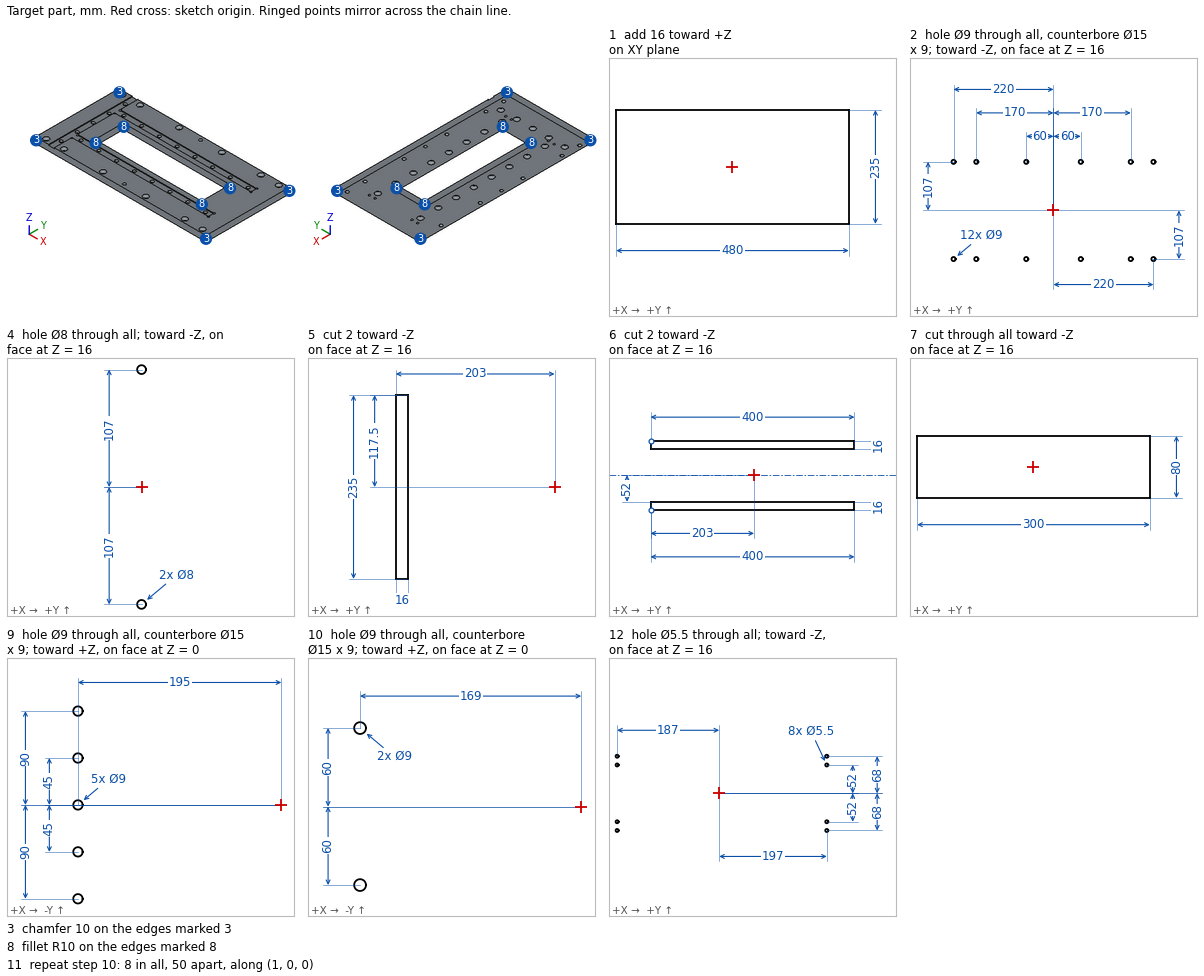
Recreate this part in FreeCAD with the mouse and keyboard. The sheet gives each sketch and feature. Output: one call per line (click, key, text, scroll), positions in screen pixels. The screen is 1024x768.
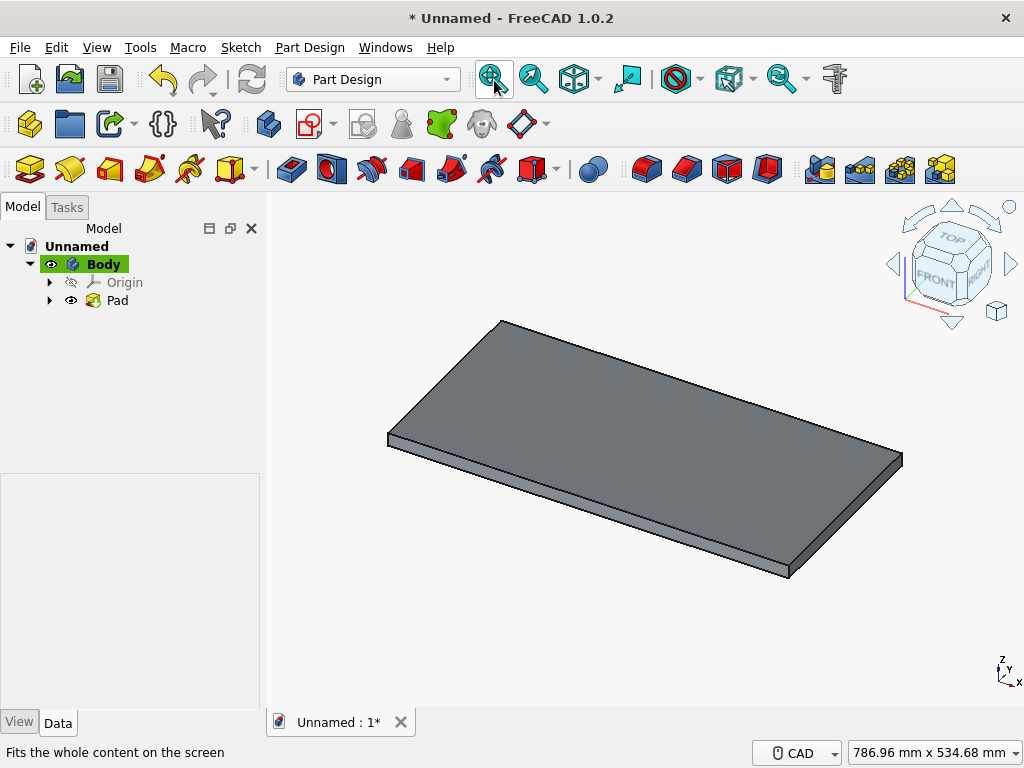
click(702, 461)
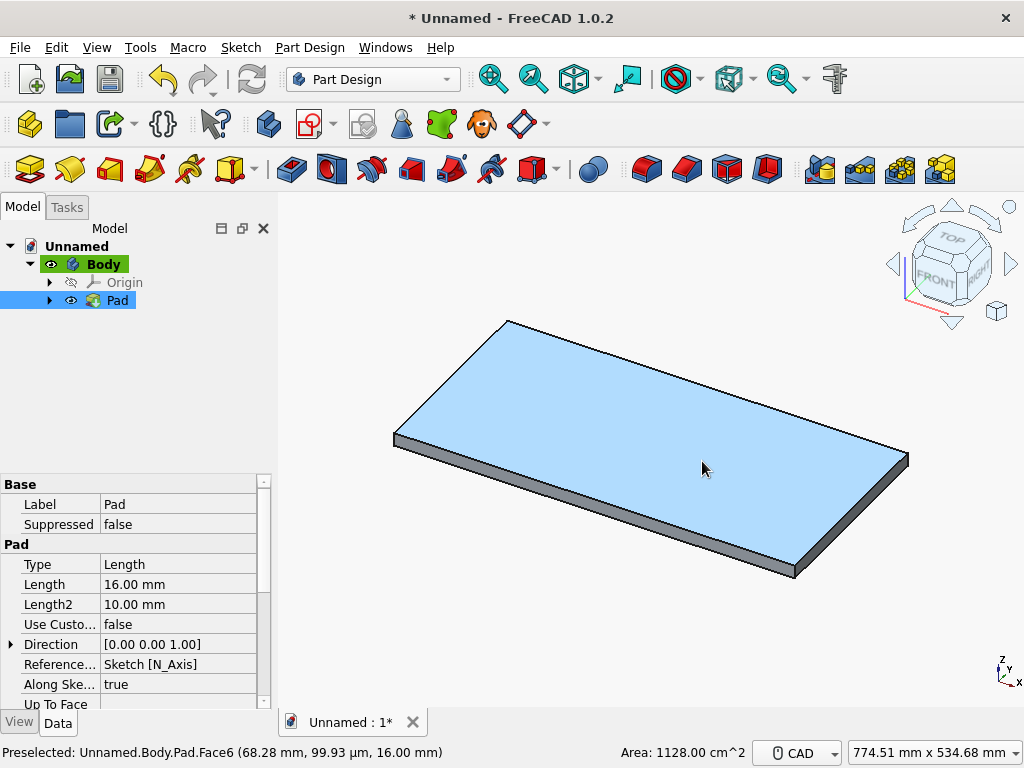
click(310, 124)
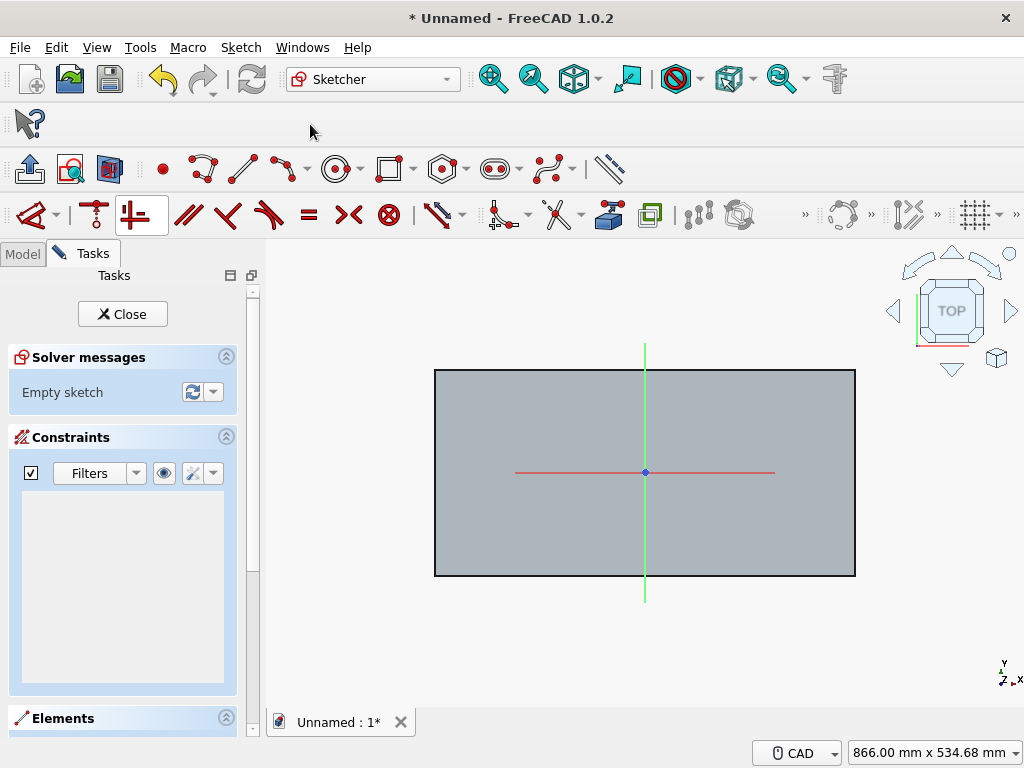
scroll(294, 473, down, 1)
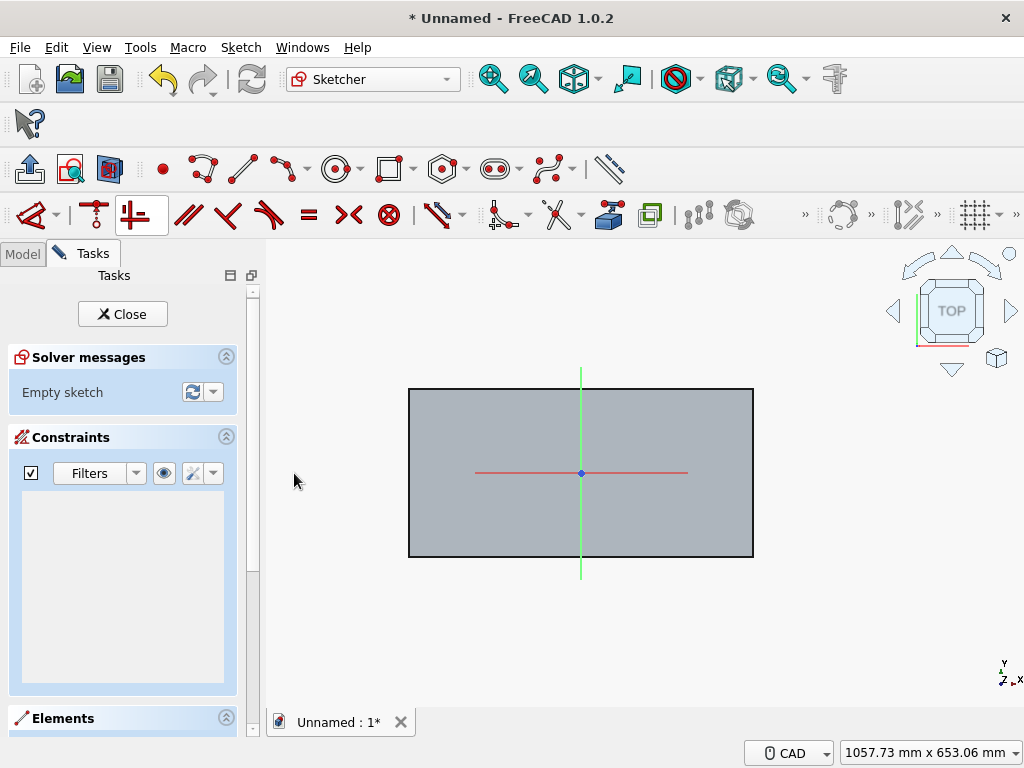
click(336, 170)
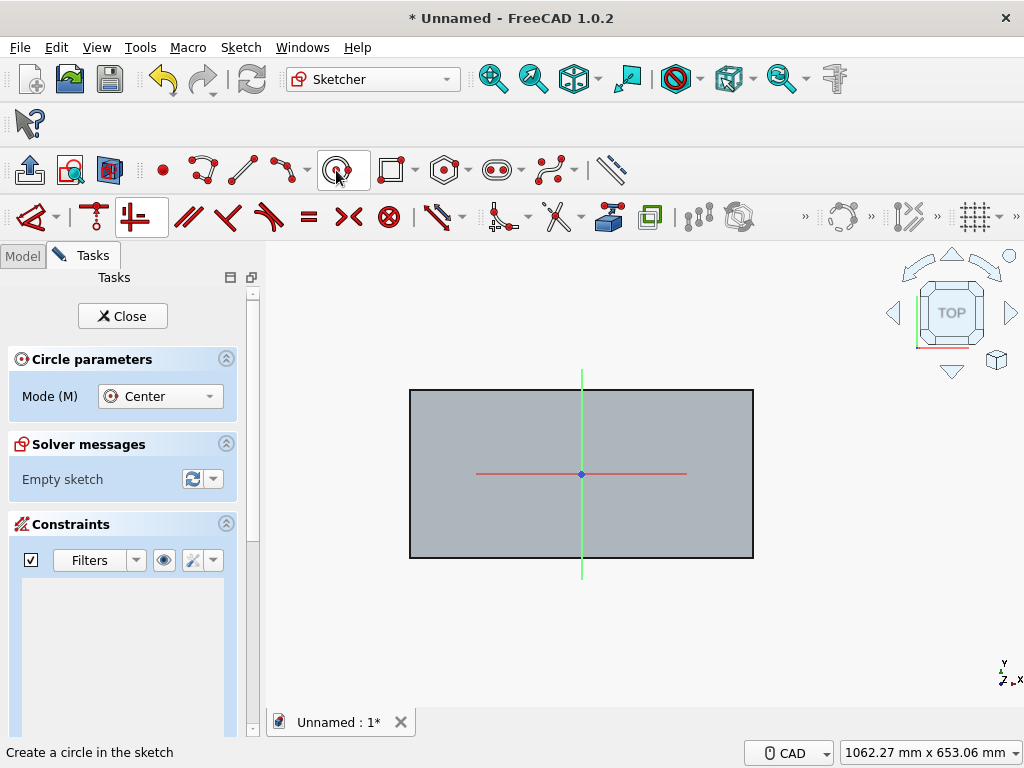
scroll(425, 398, up, 10)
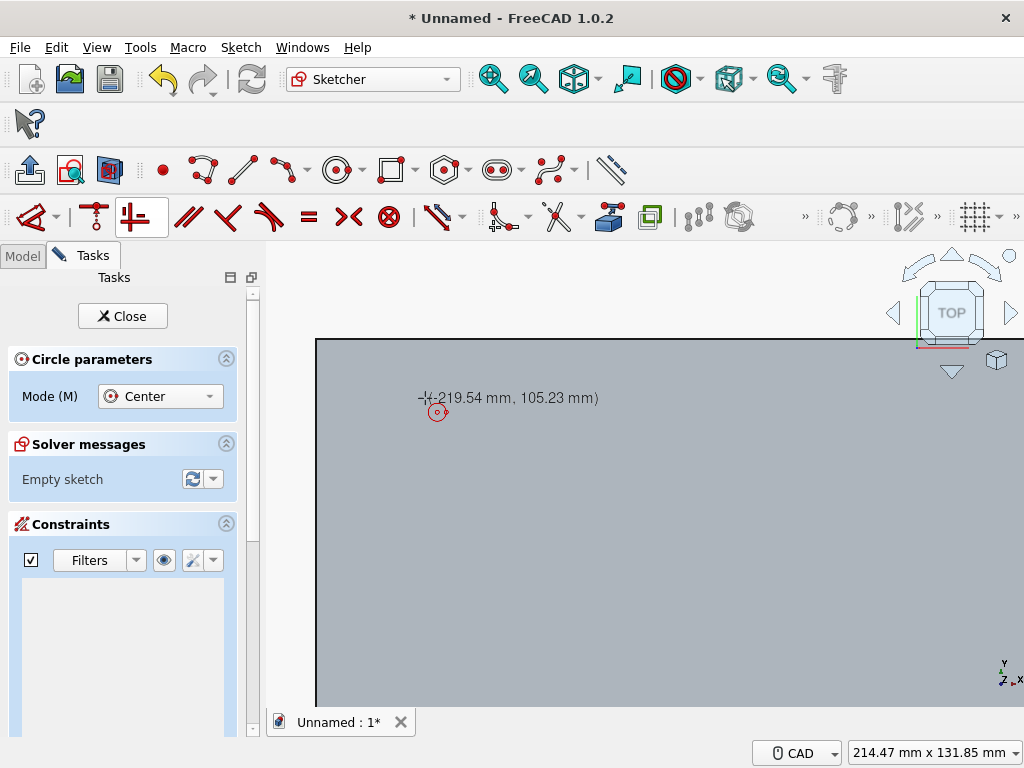
scroll(378, 378, down, 9)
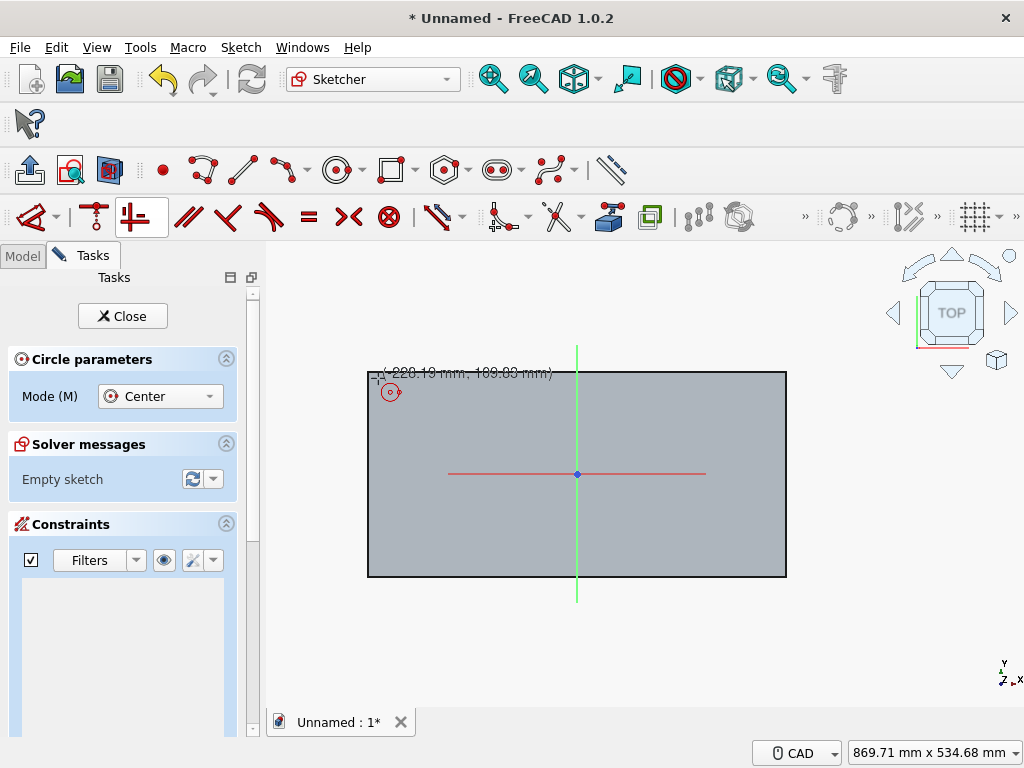
click(385, 381)
move(388, 378)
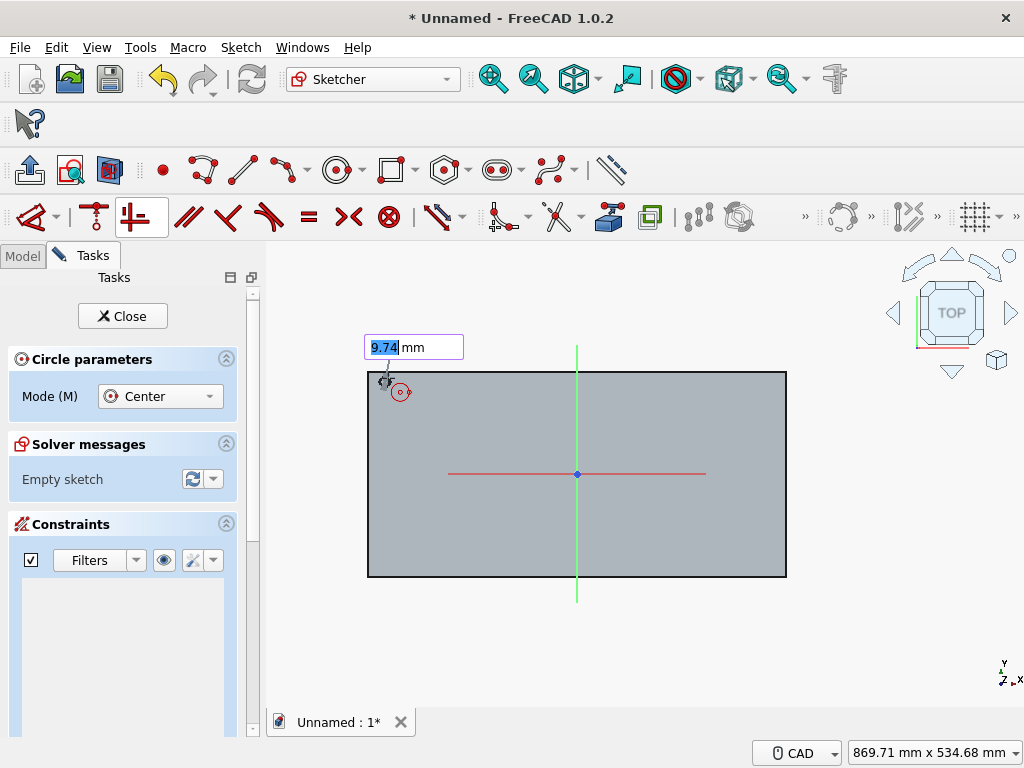
text(9)
key(Return)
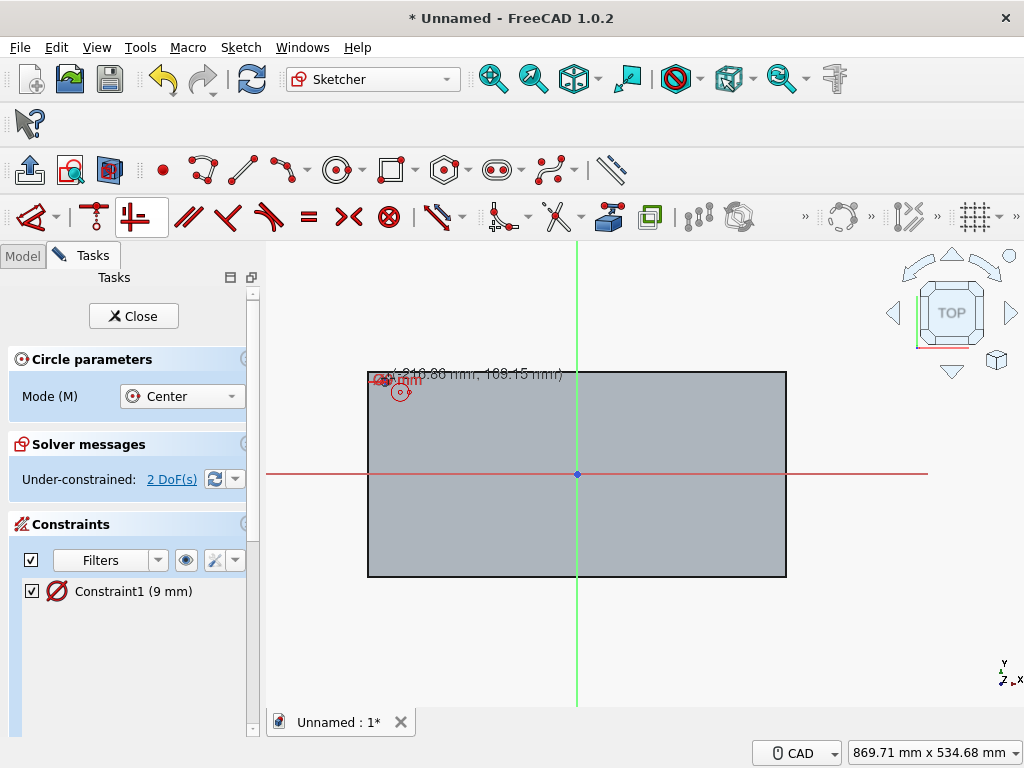
scroll(769, 567, up, 9)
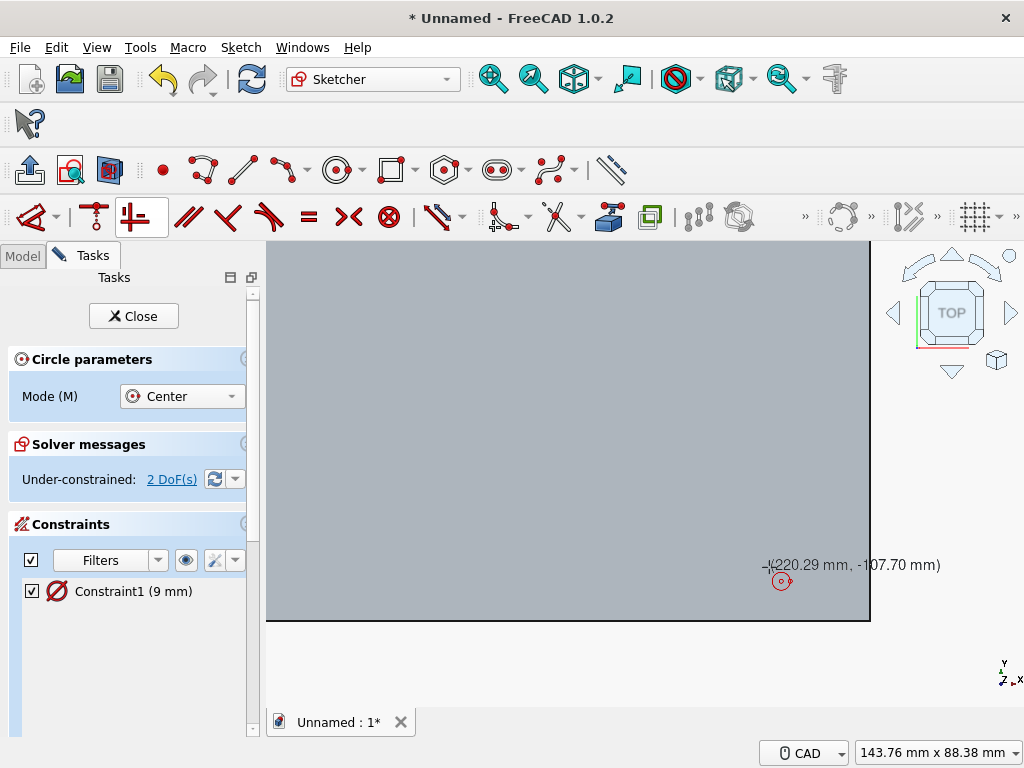
scroll(769, 568, down, 9)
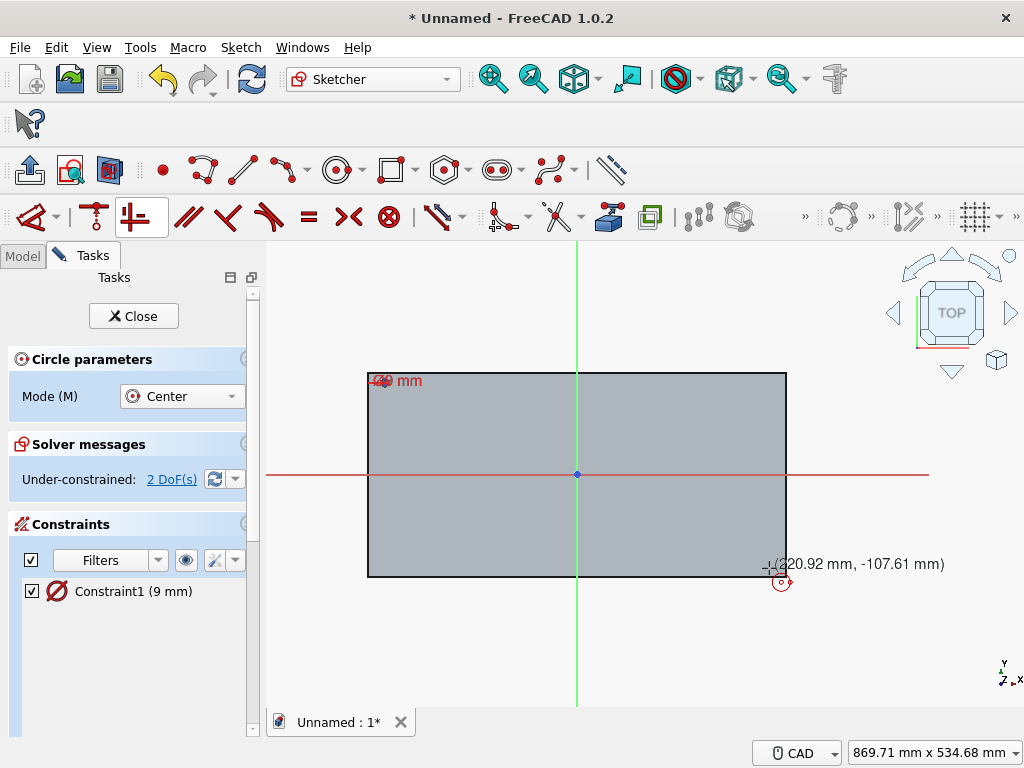
click(769, 568)
move(772, 565)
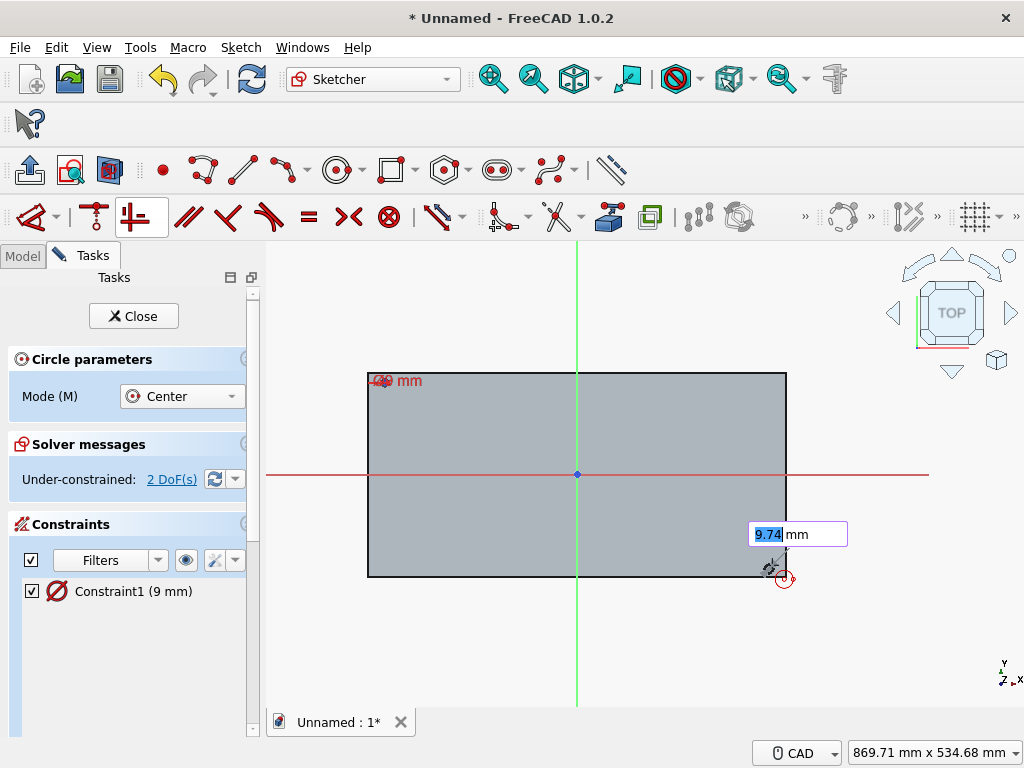
text(9)
key(Return)